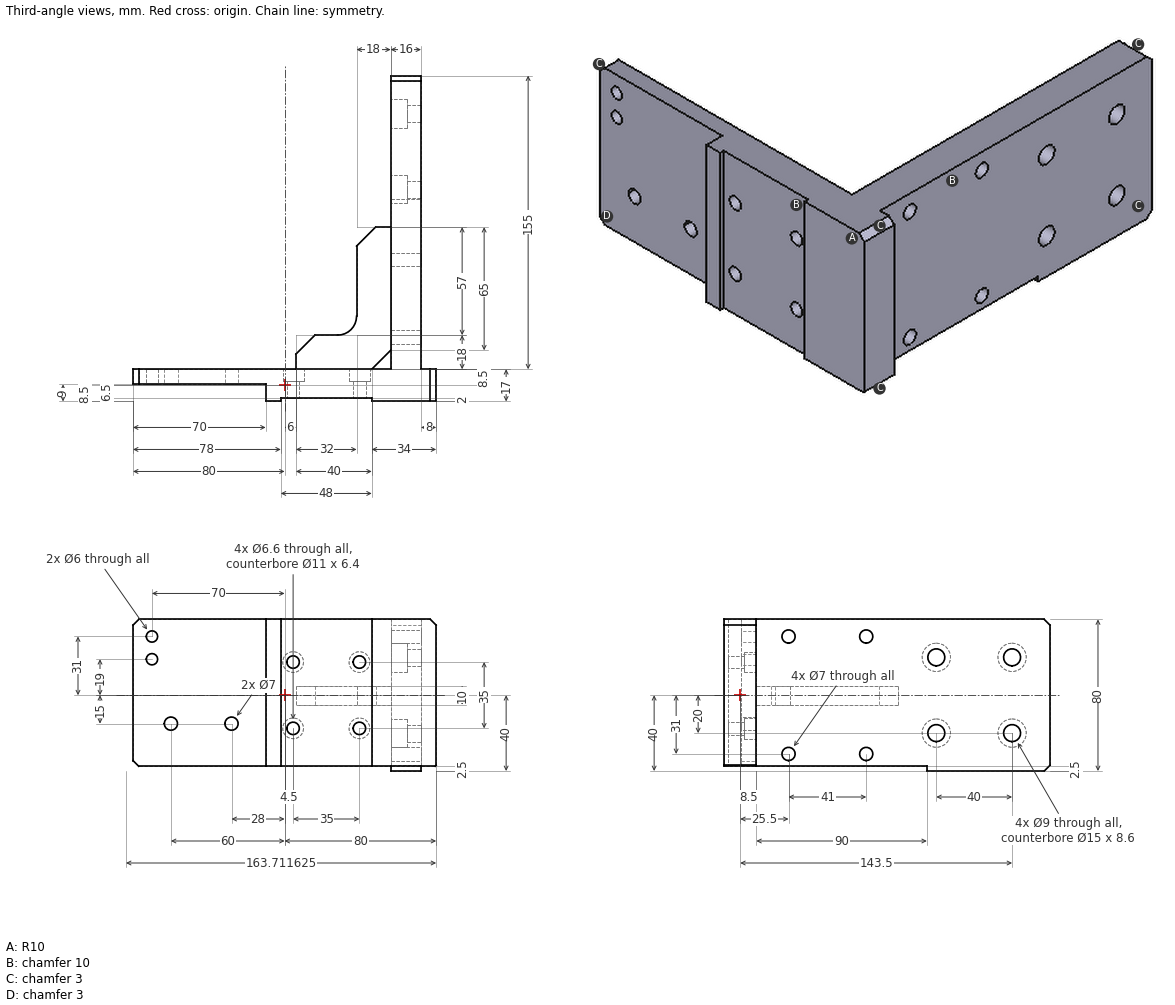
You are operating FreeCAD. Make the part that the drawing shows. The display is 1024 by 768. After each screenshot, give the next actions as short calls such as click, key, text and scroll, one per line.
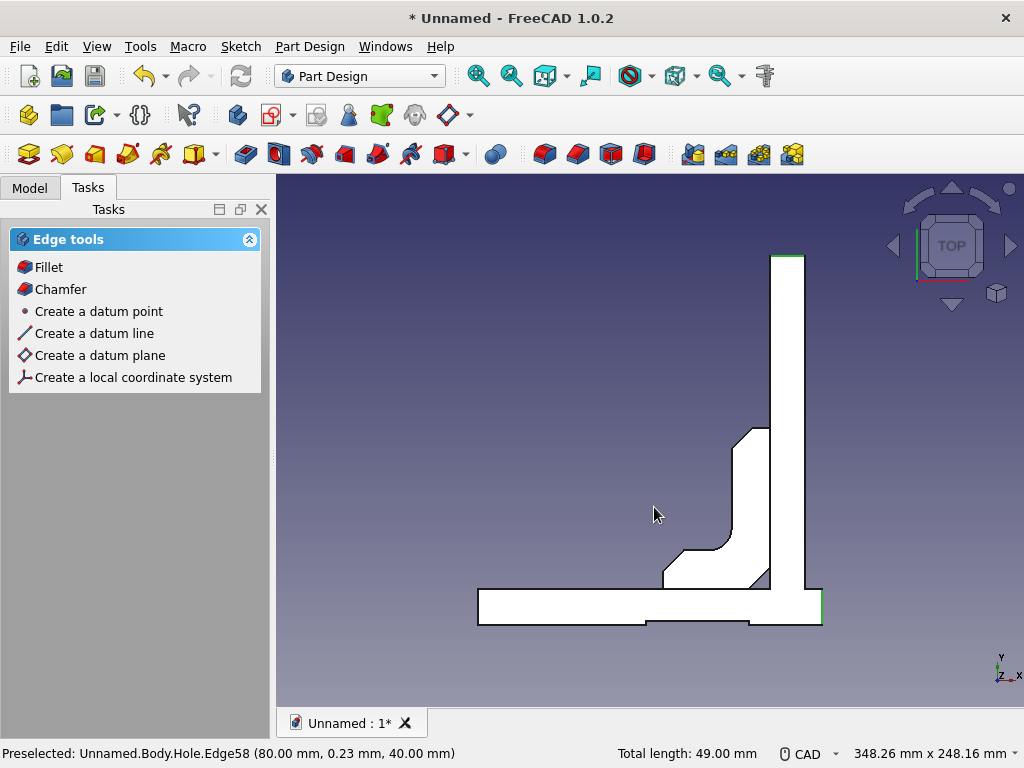
click(478, 606, ctrl)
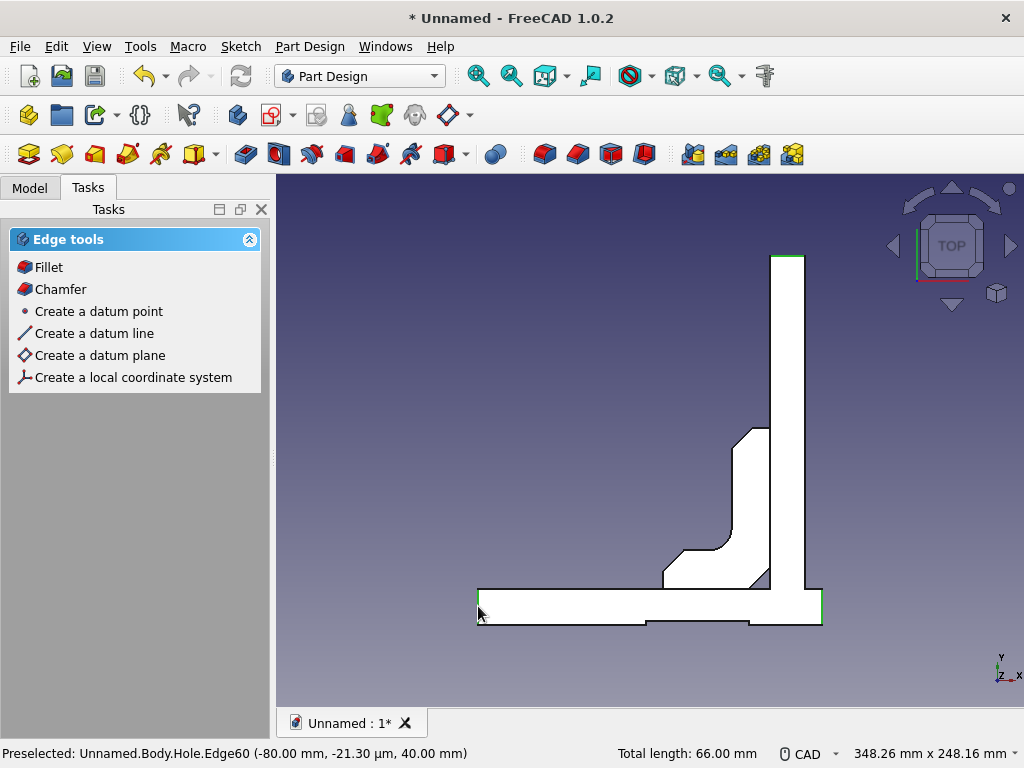
key(1)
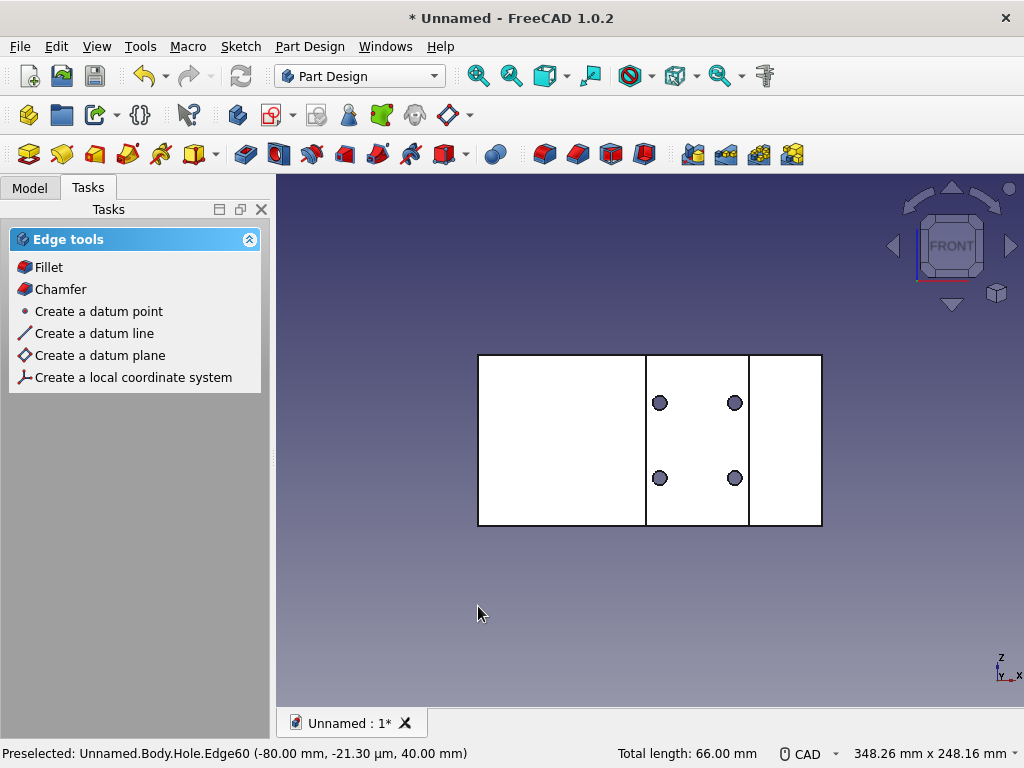
key(3)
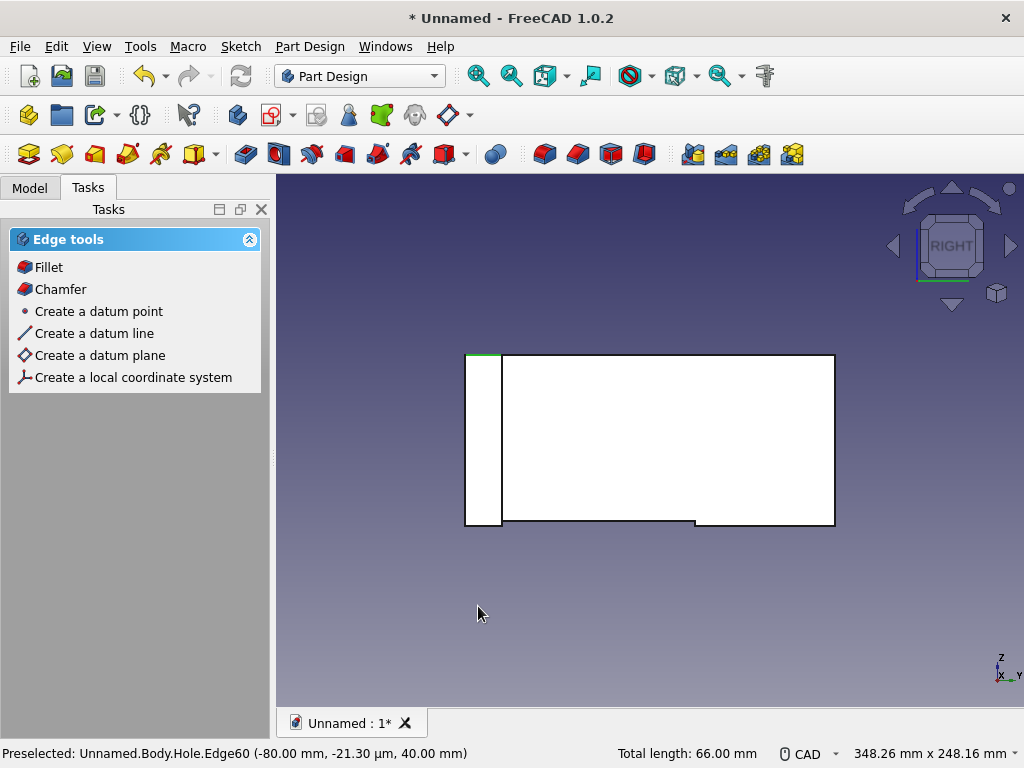
click(484, 525, ctrl)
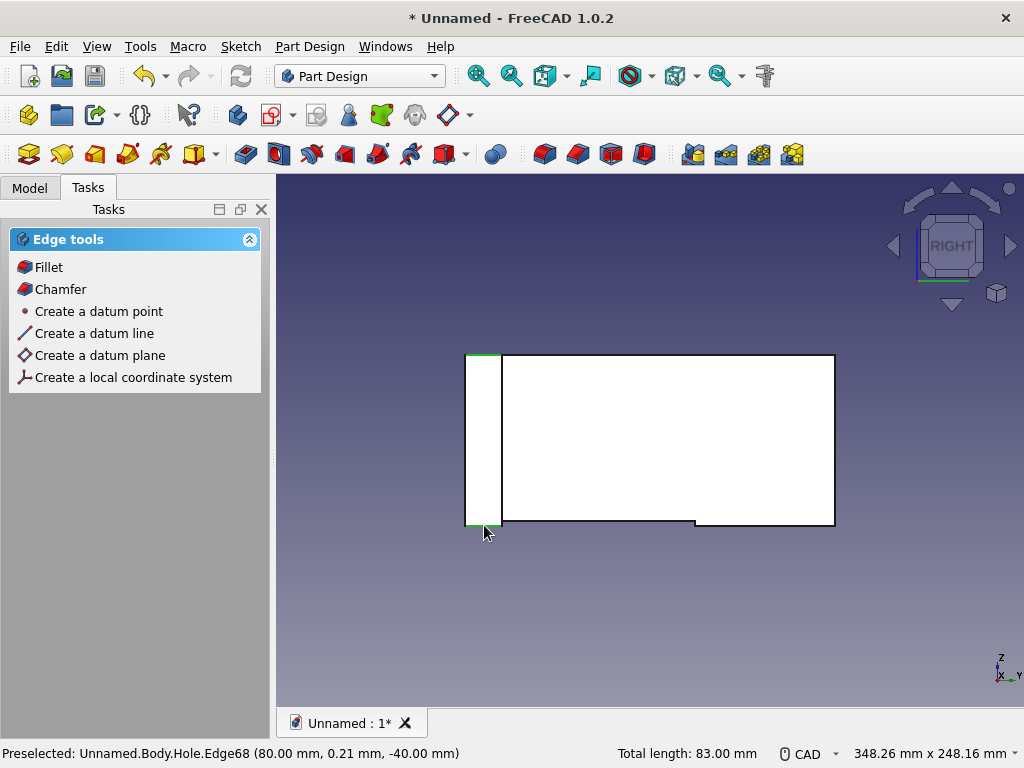
click(578, 154)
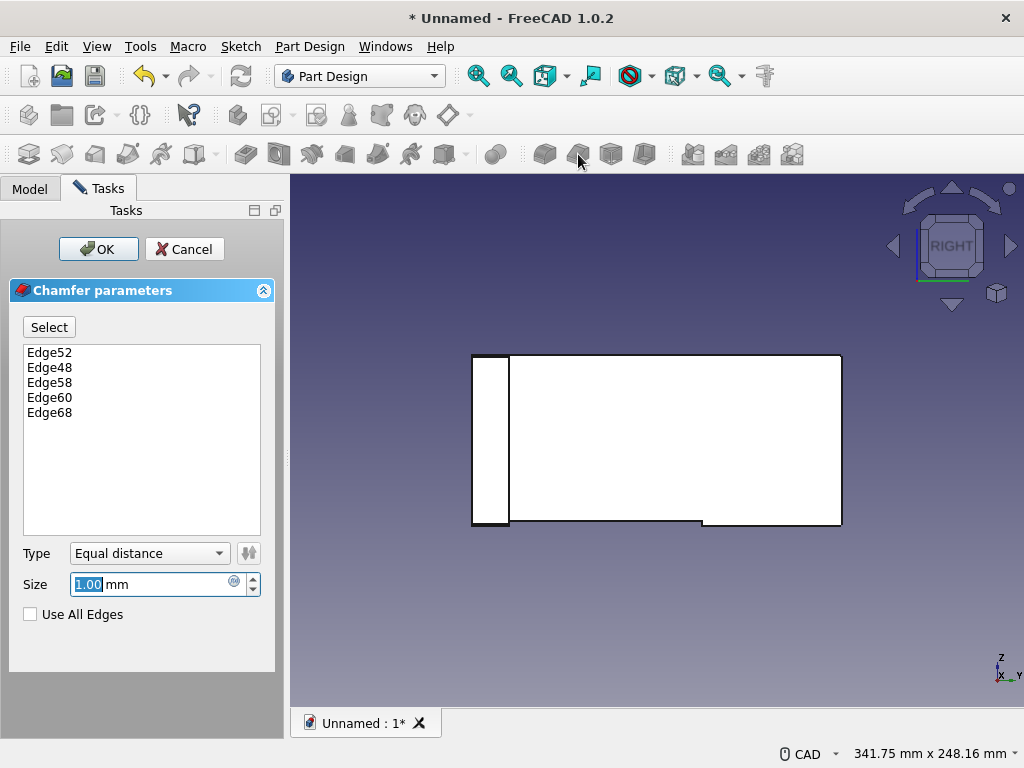
text(3)
key(Tab)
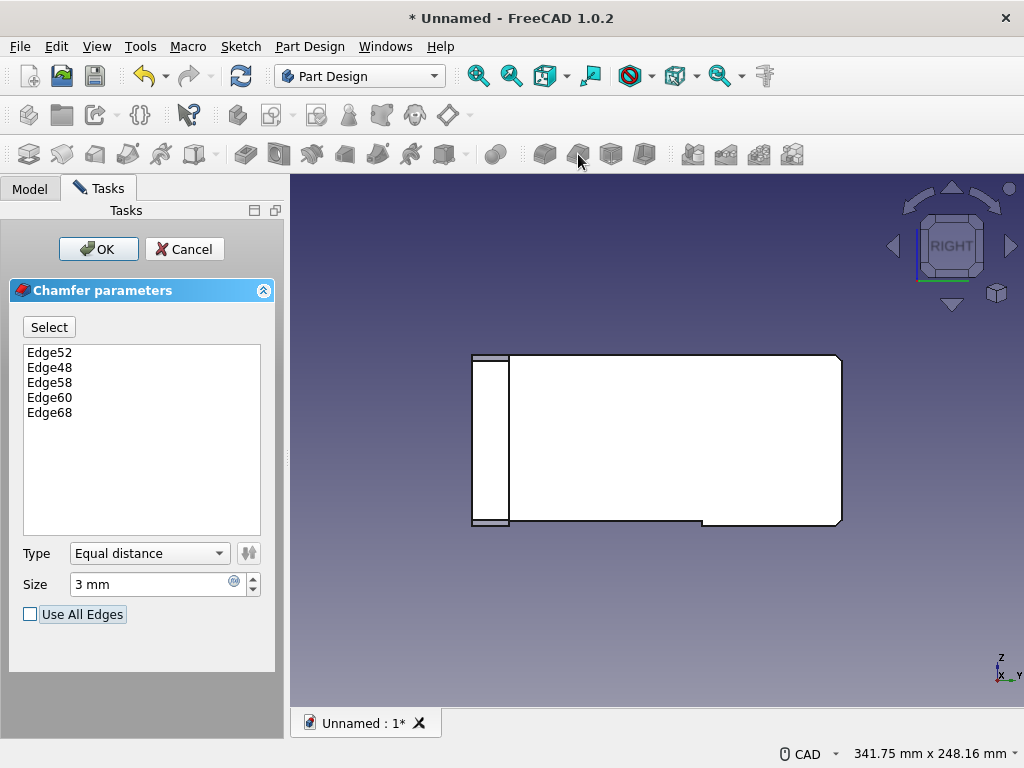
click(99, 249)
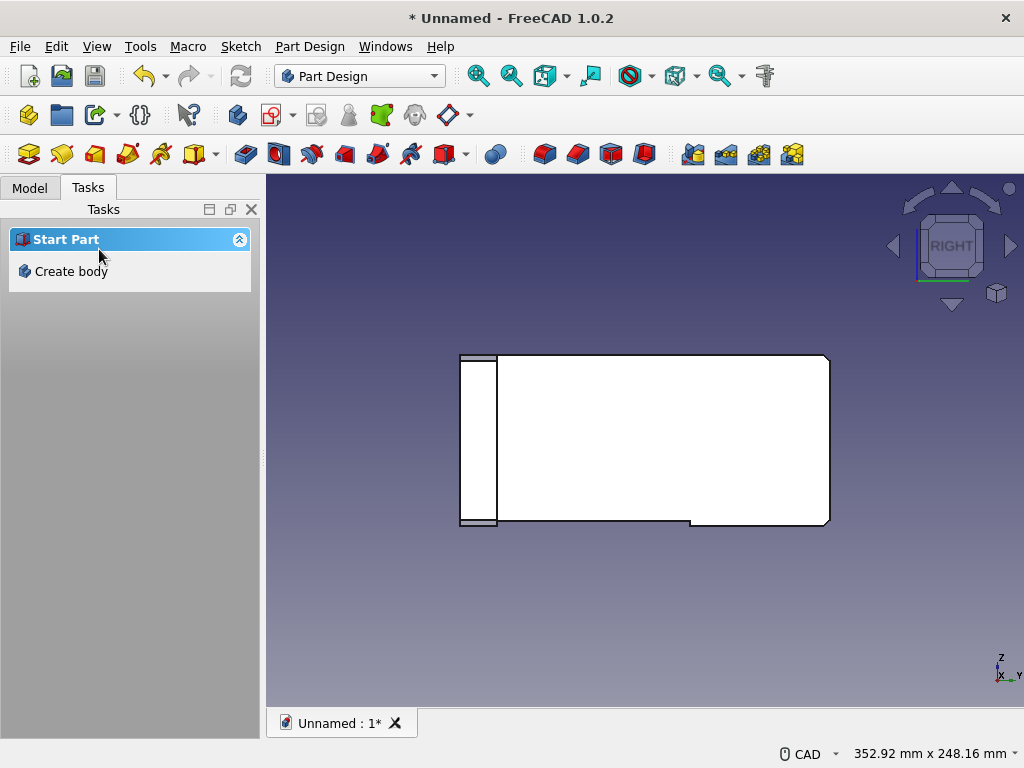
key(6)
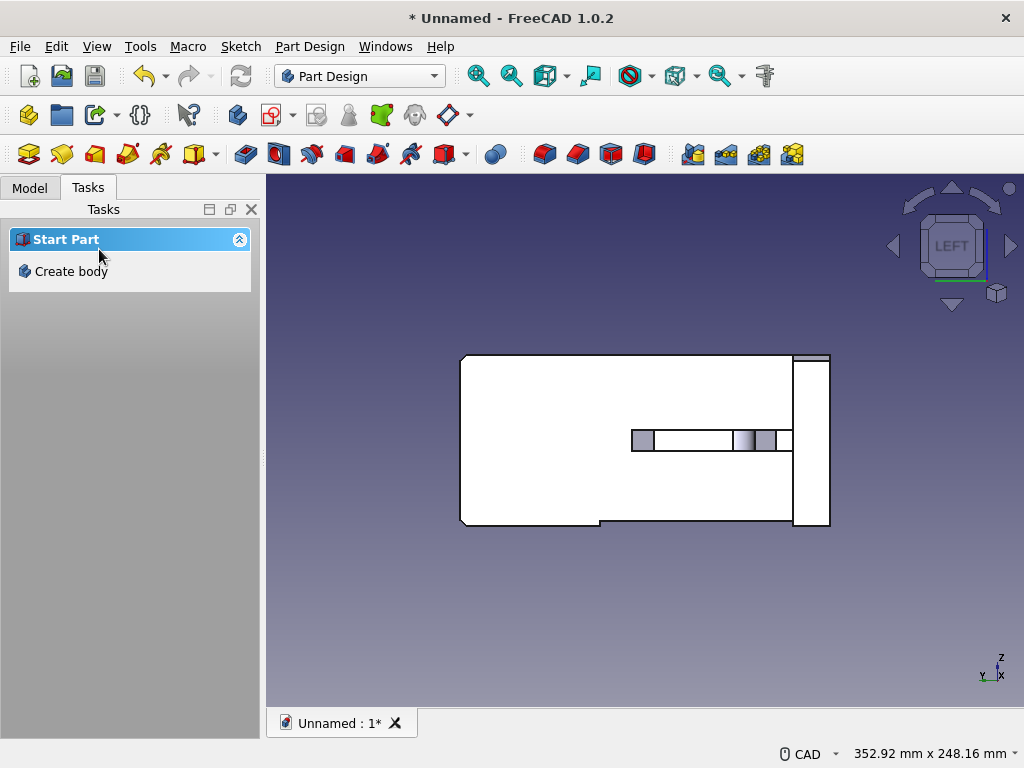
click(532, 440)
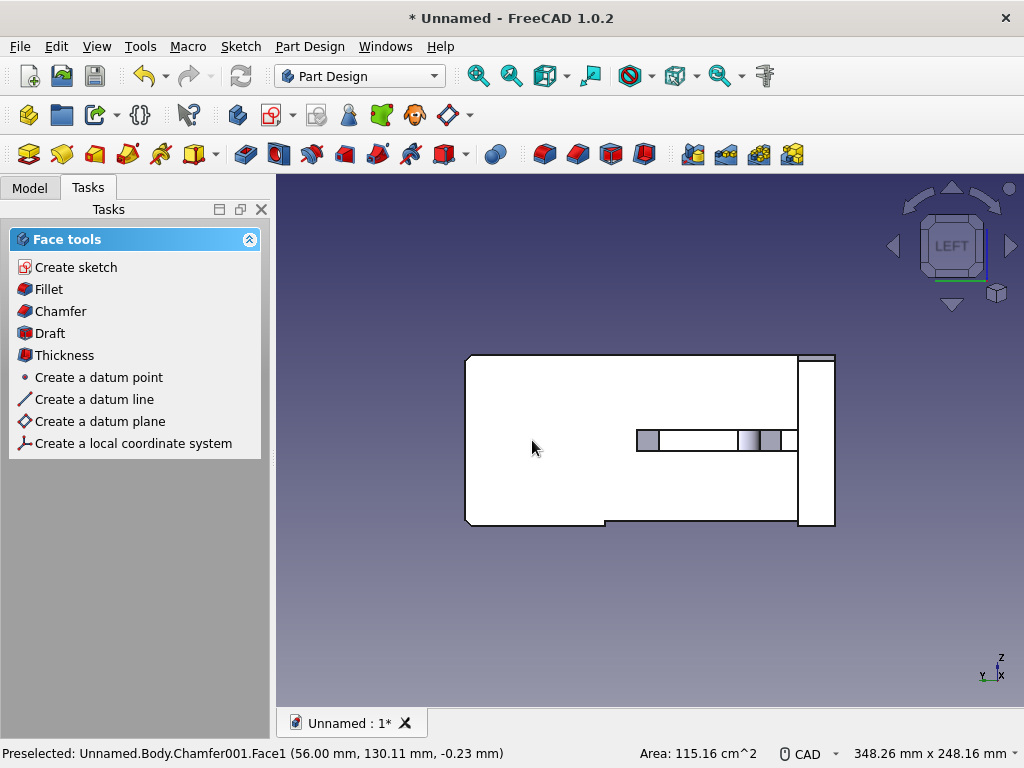
click(270, 116)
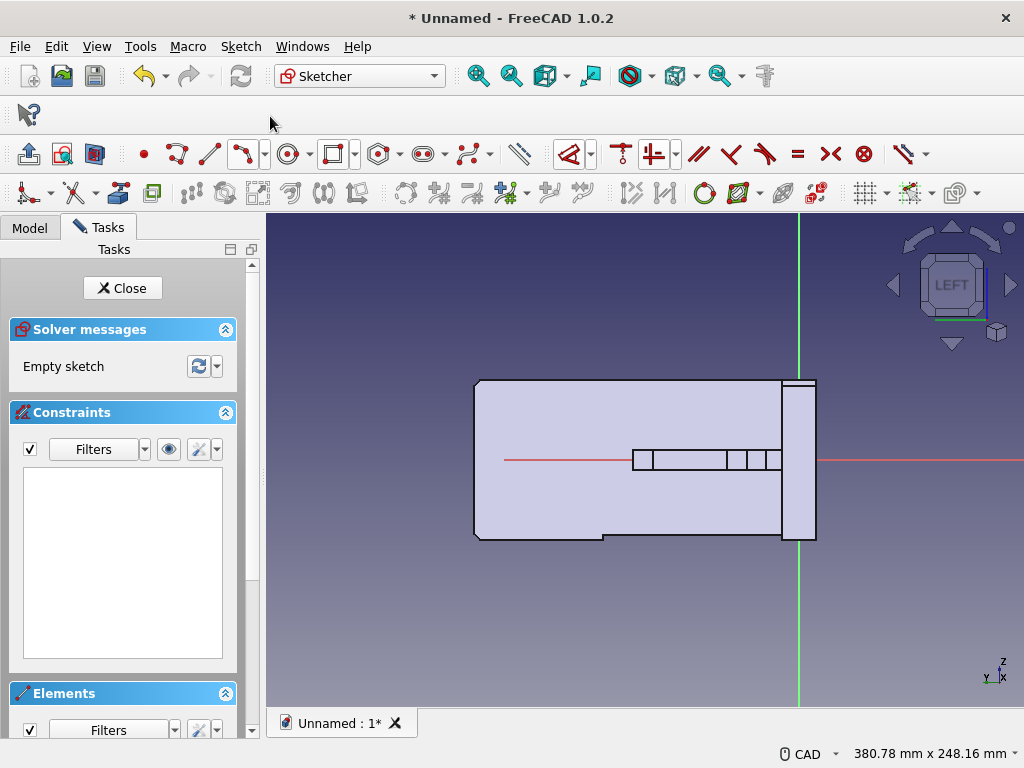
key(q)
key(s)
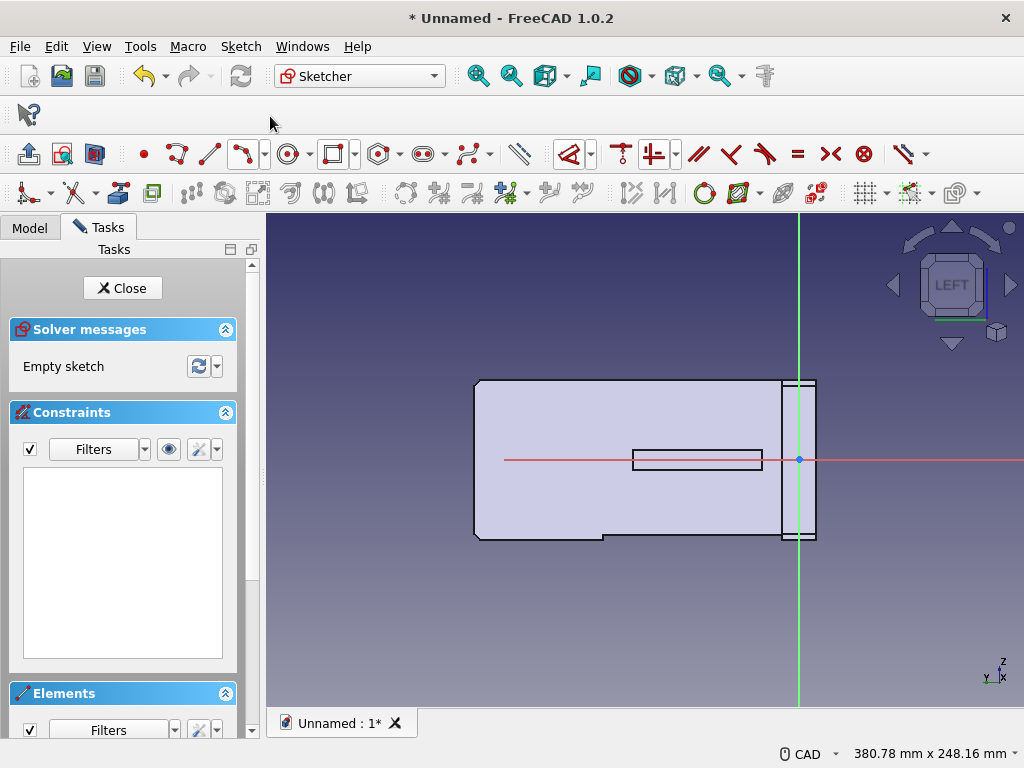
scroll(855, 460, up, 4)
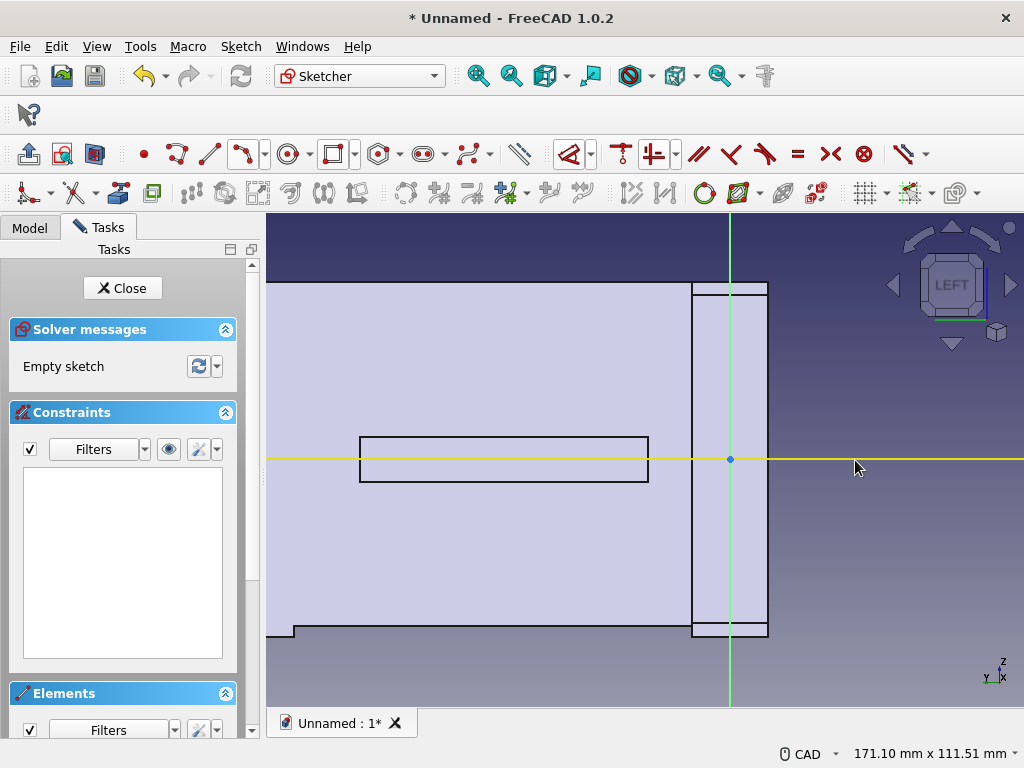
click(288, 154)